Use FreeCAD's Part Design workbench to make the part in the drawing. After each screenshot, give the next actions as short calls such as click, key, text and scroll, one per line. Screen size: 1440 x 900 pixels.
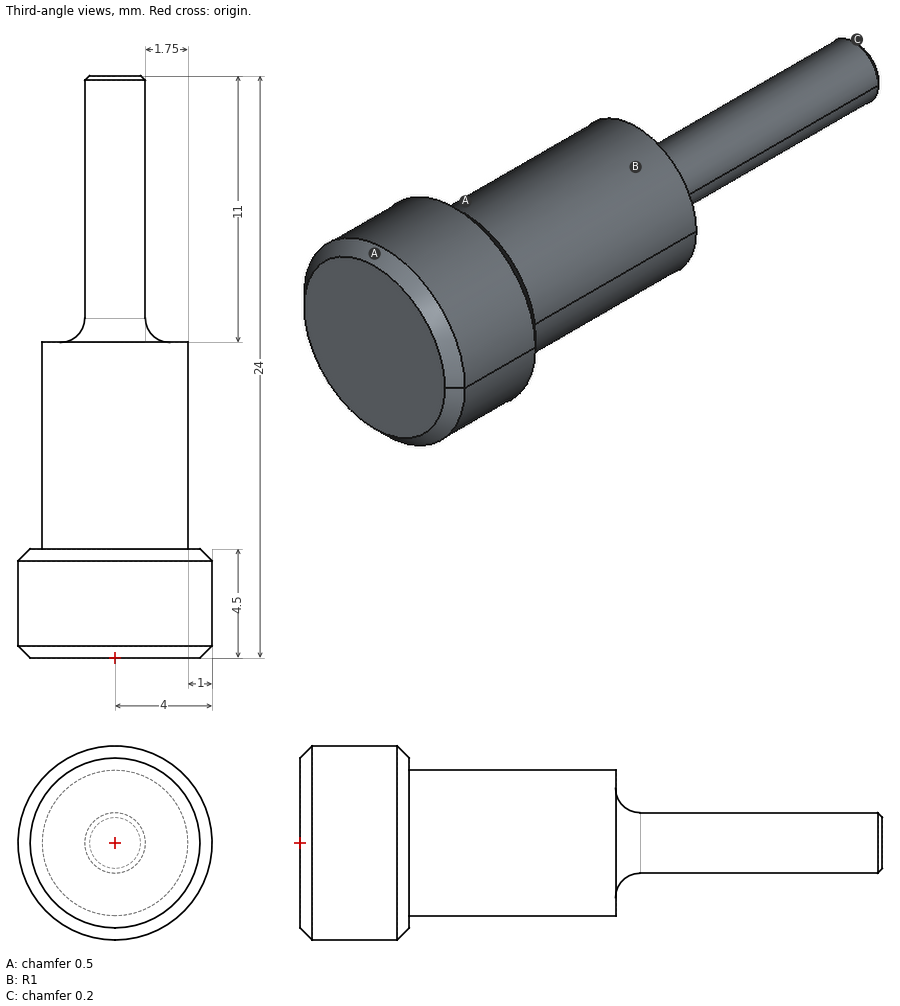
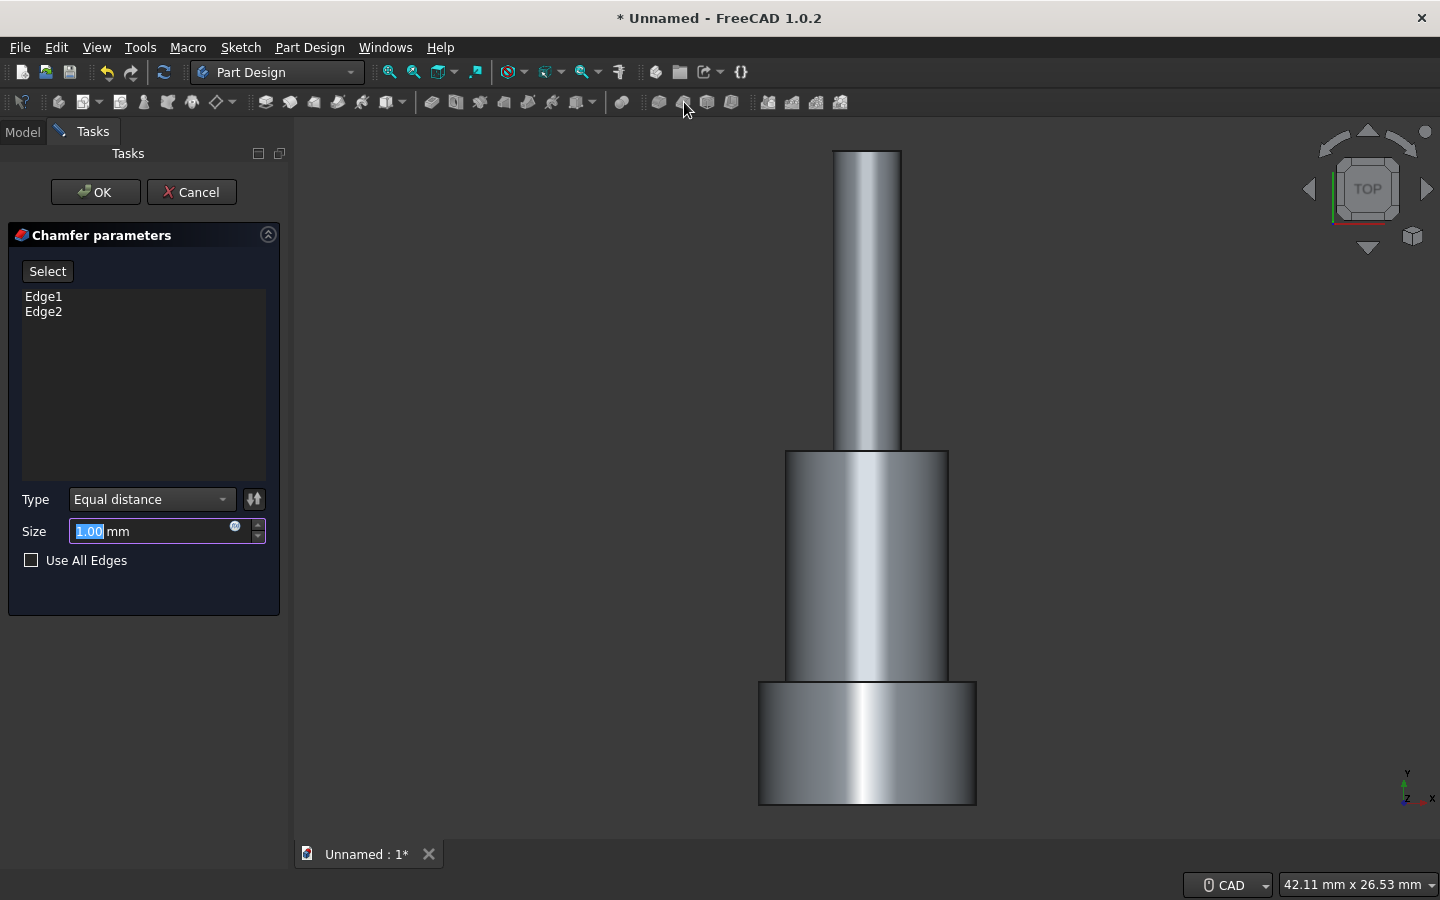
text(0.5)
key(Tab)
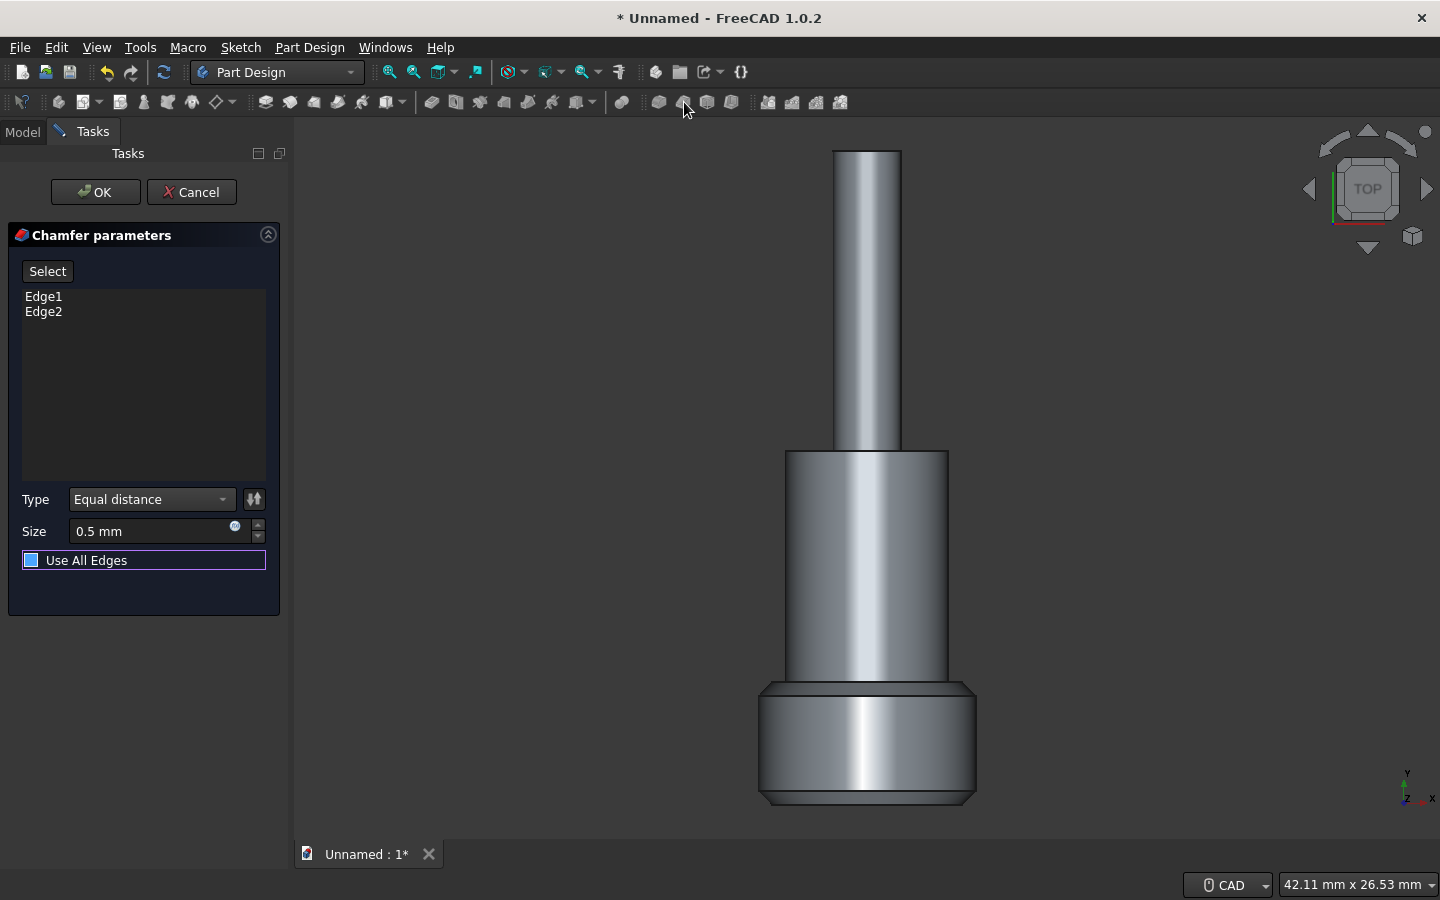
click(96, 192)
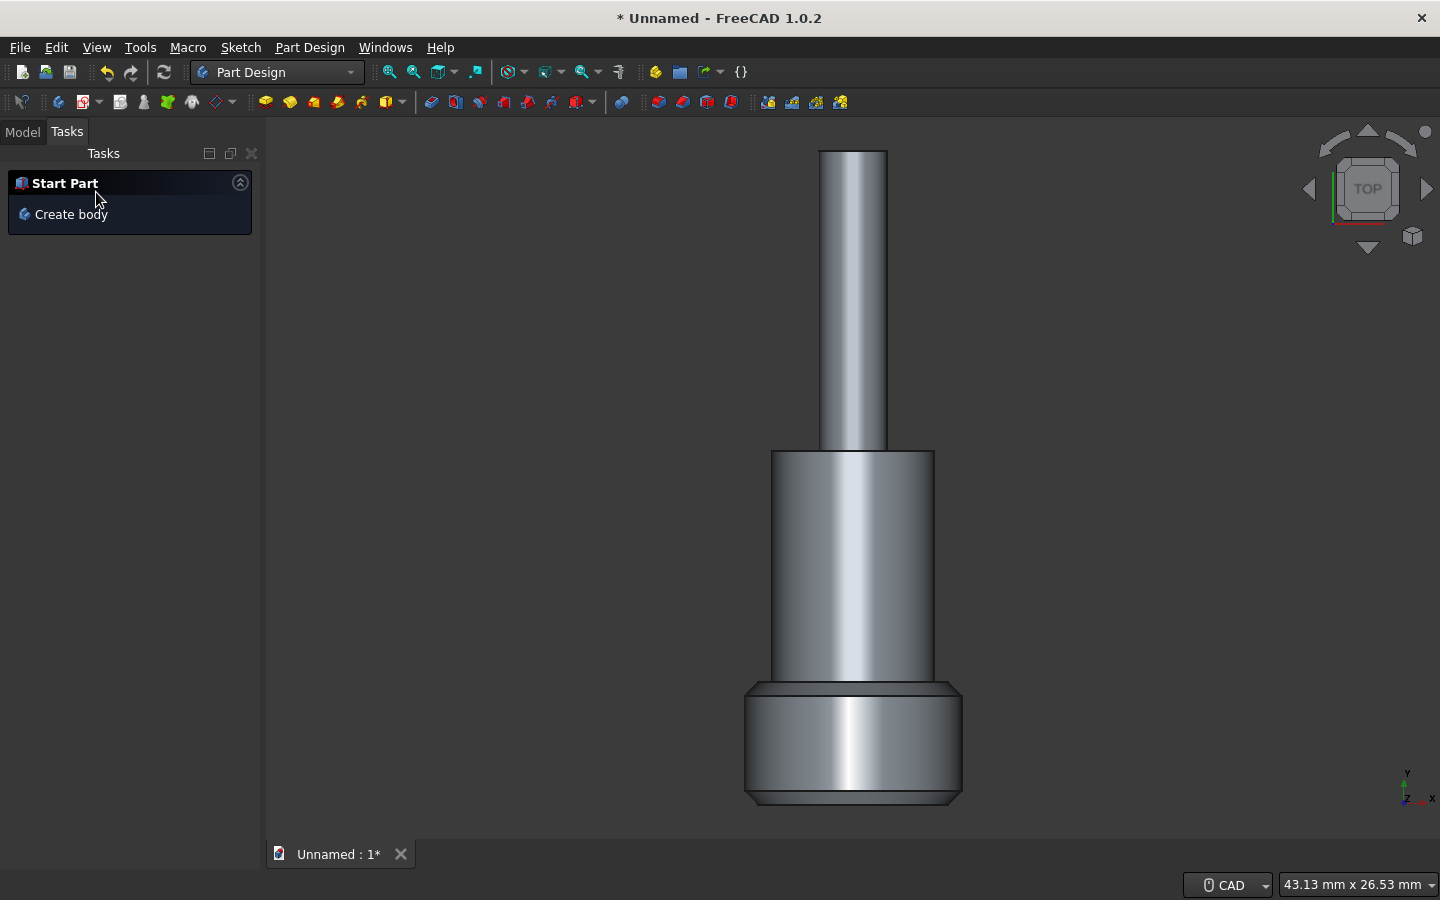
key(0)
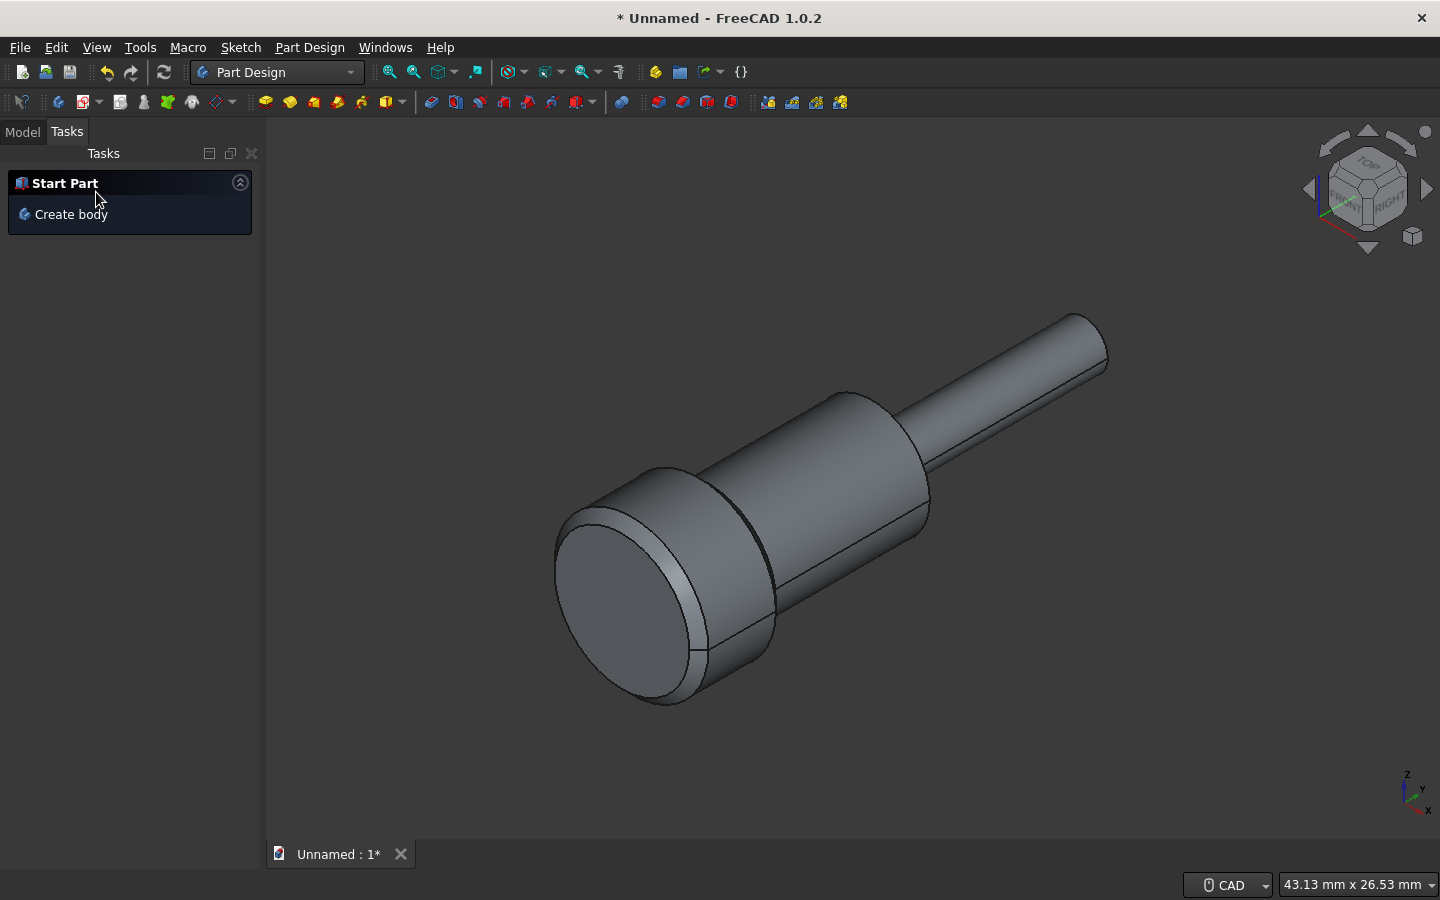
key(2)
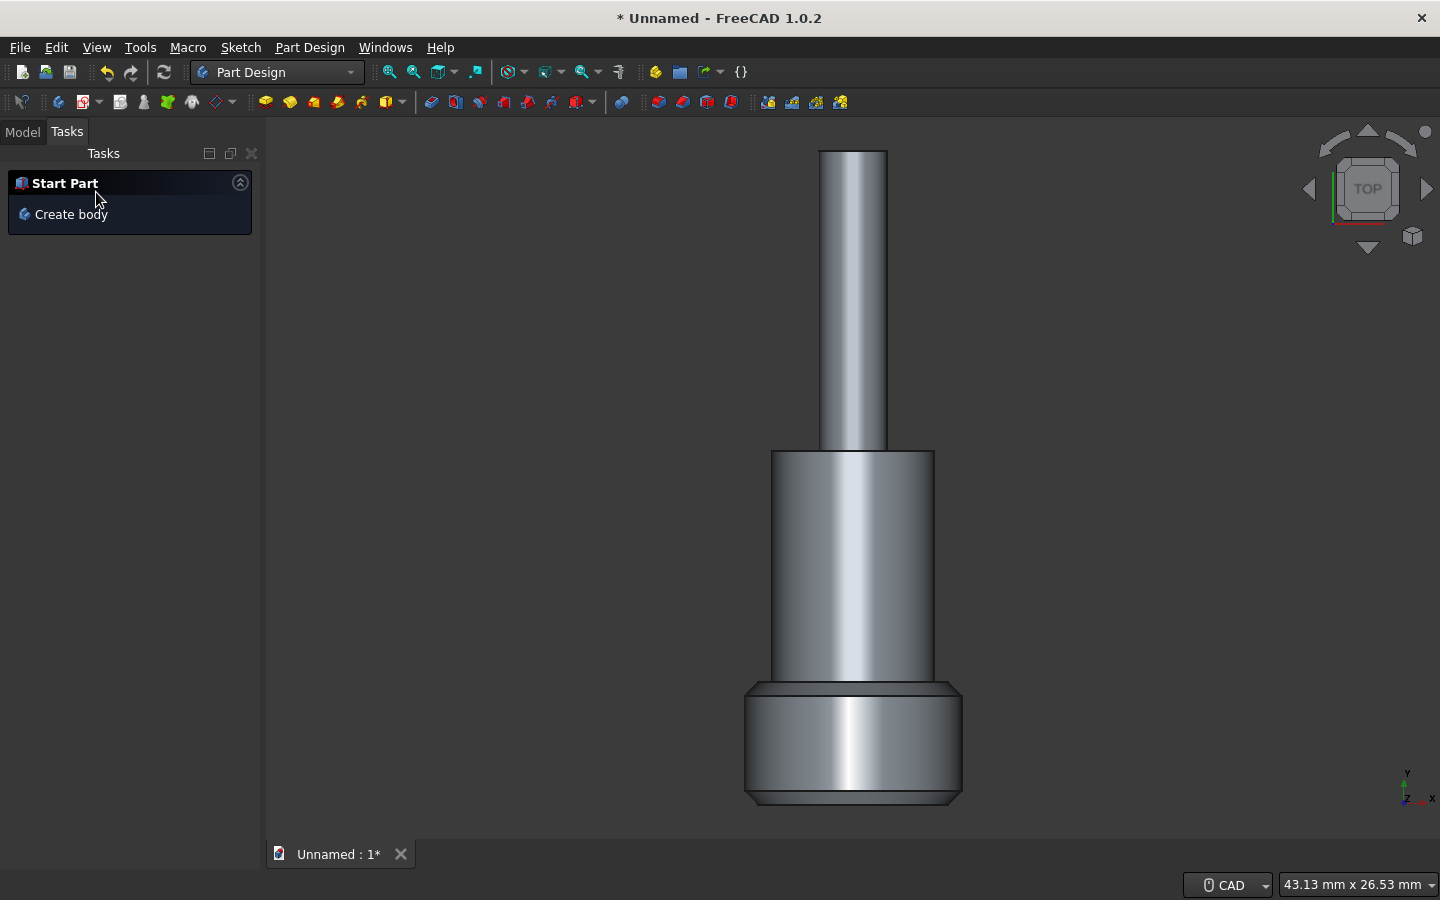
key(1)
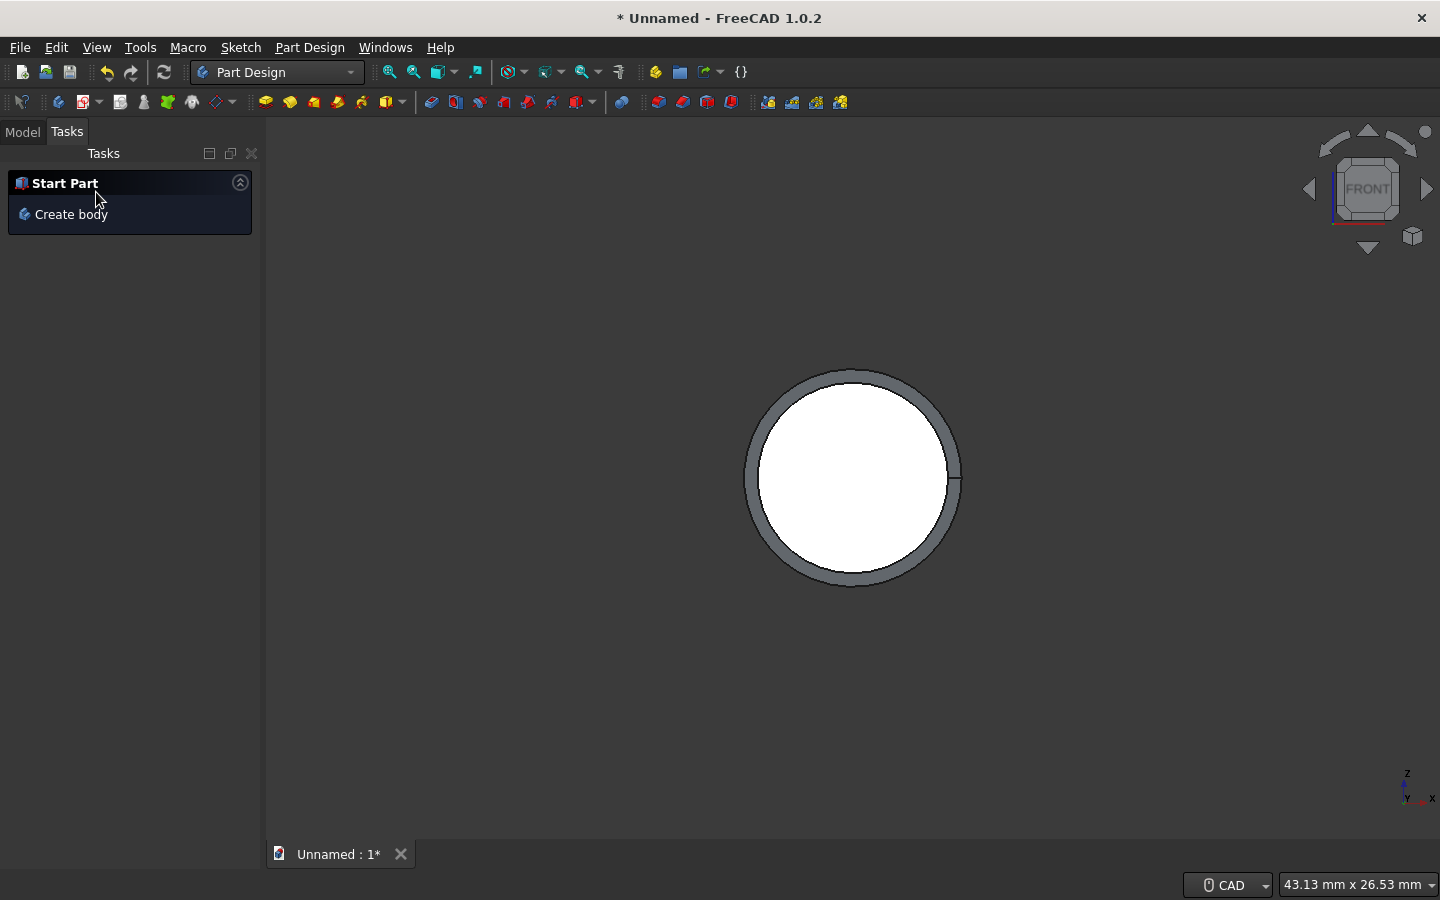
click(390, 72)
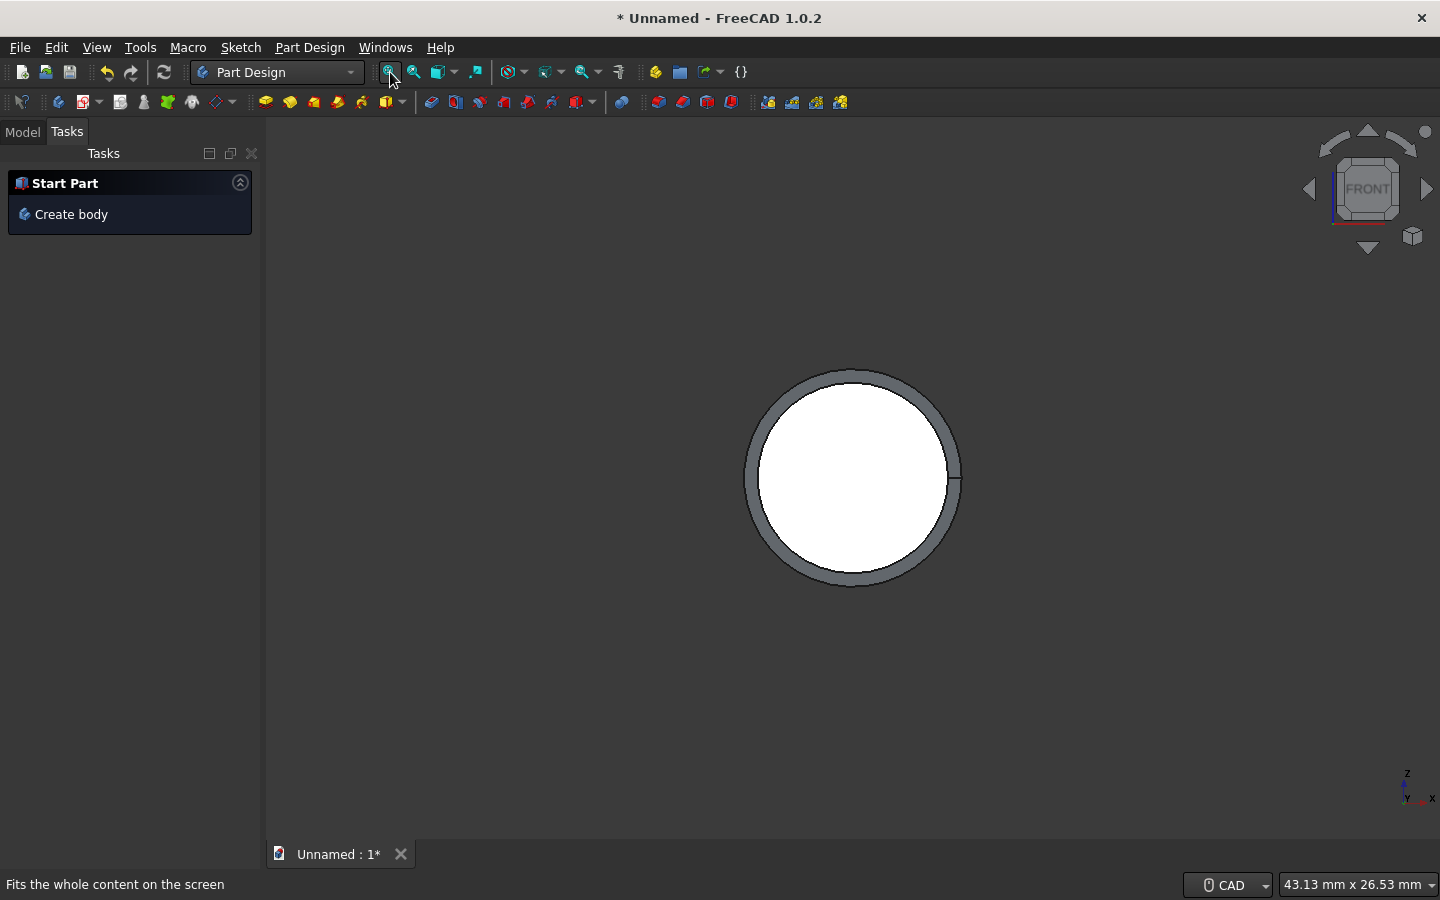
key(3)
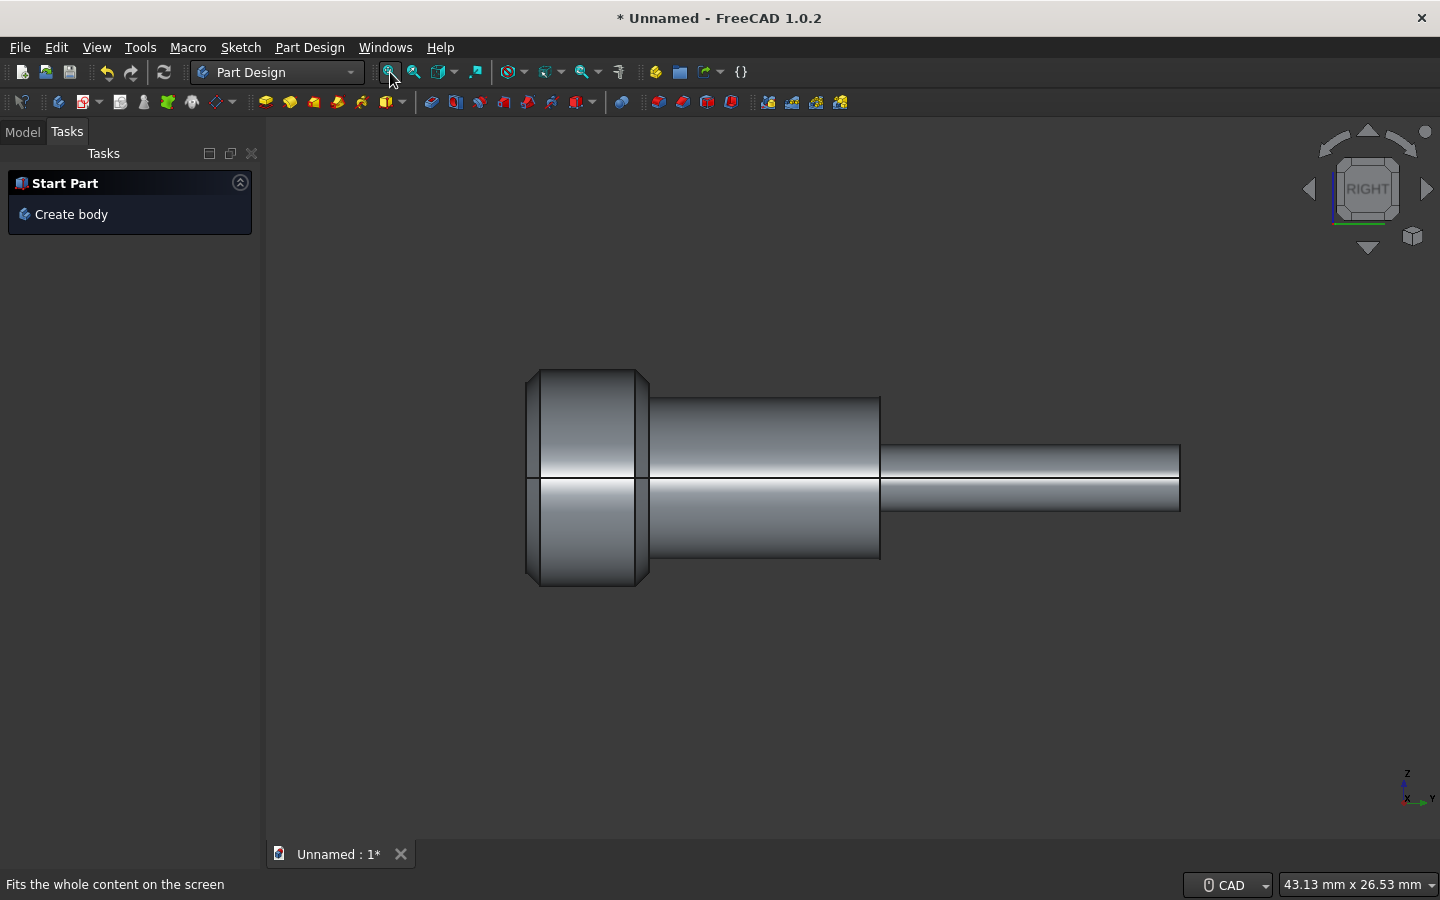
key(5)